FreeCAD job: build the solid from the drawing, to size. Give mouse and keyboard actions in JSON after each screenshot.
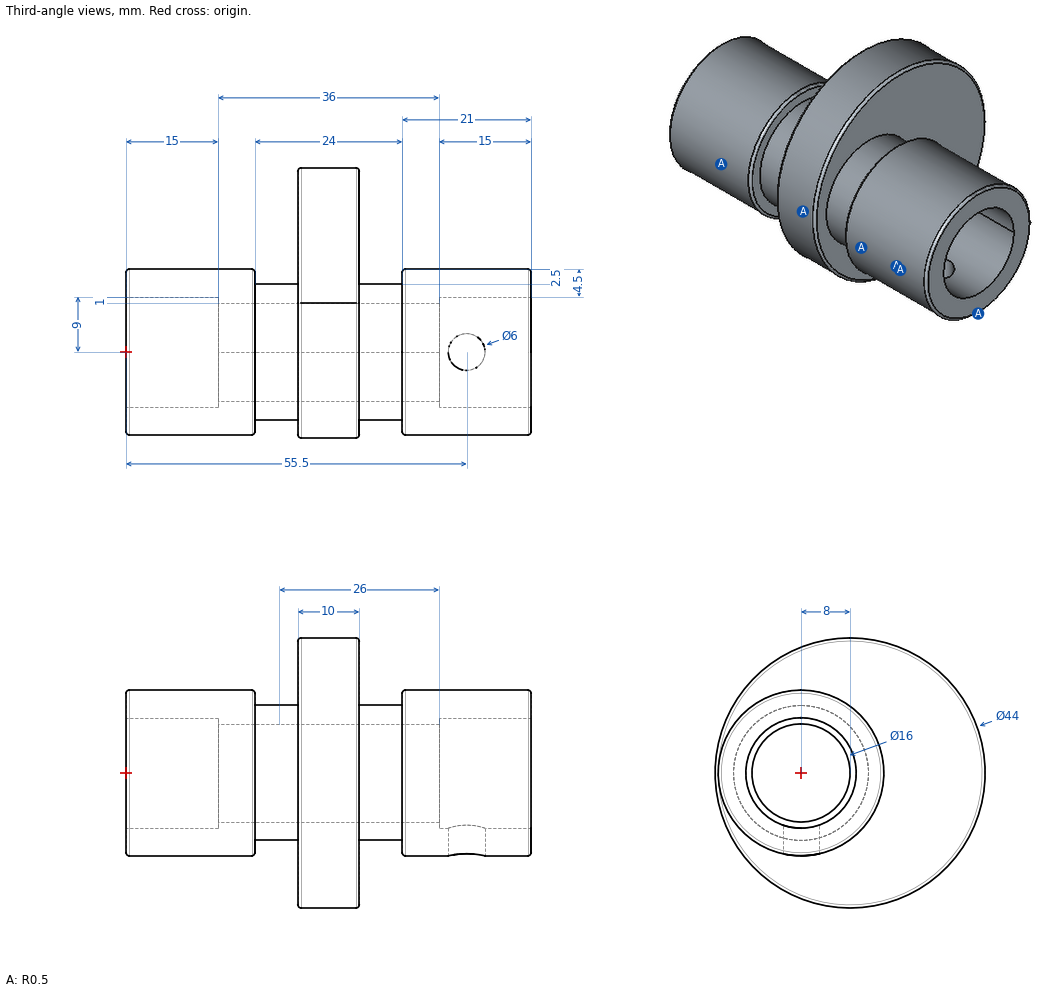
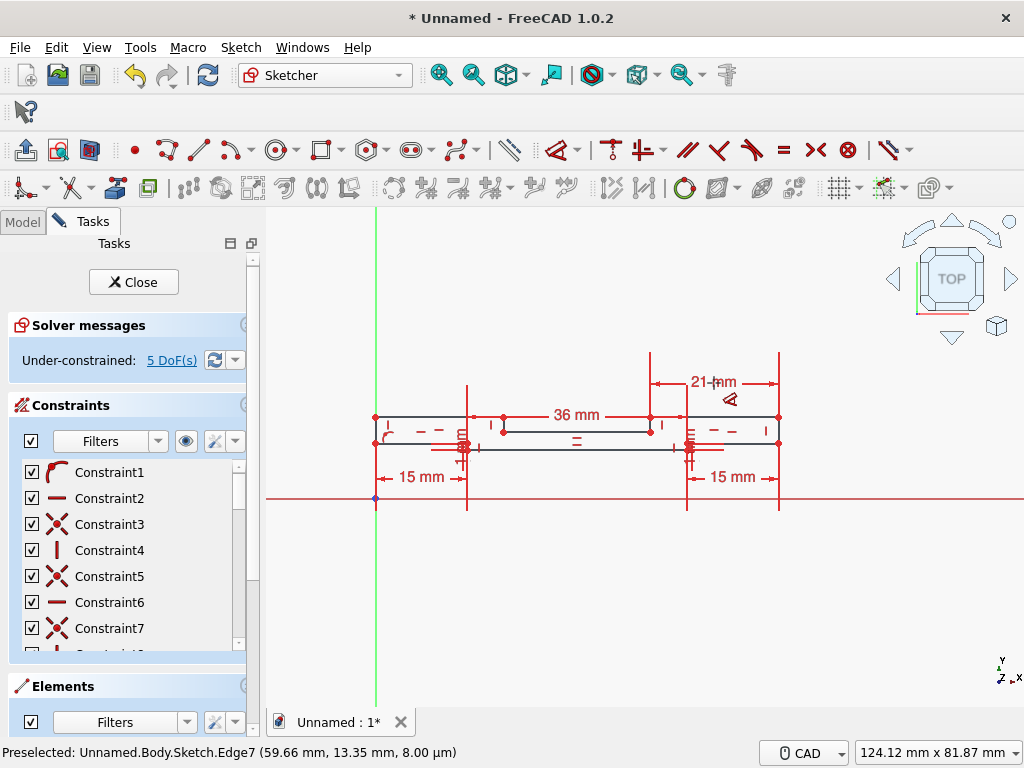
{"action": "left_click", "coordinate": [606, 432]}
{"action": "left_click", "coordinate": [577, 466]}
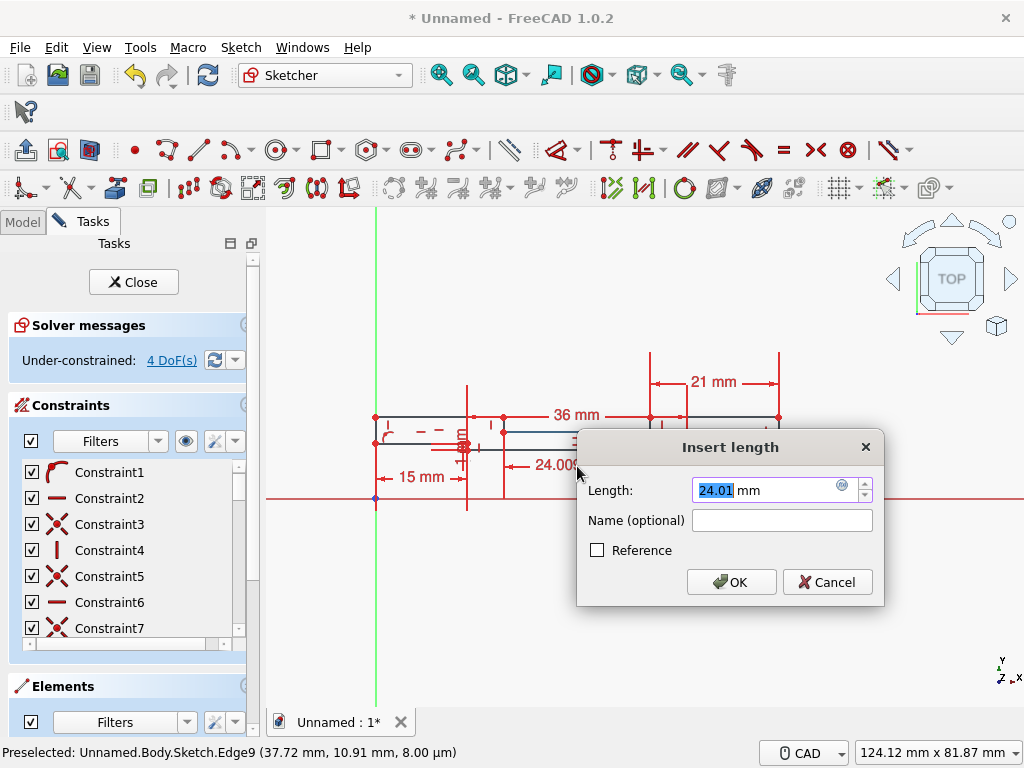
{"action": "type", "text": "24"}
{"action": "key", "text": "Return"}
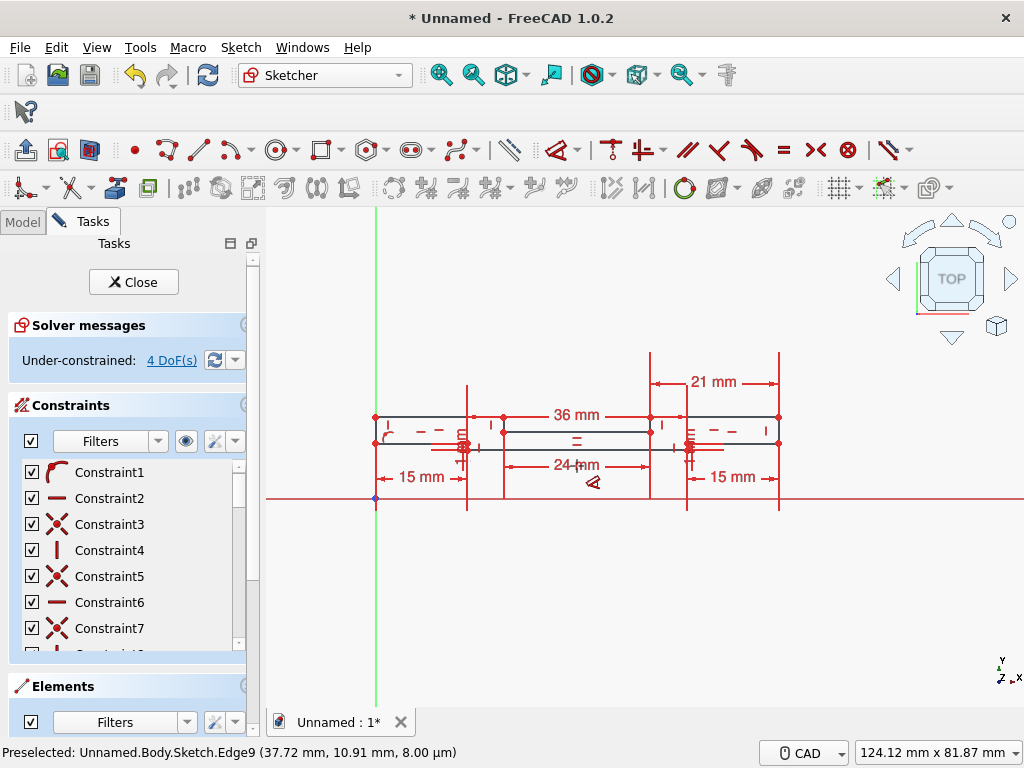
{"action": "left_click", "coordinate": [376, 444]}
{"action": "left_click", "coordinate": [342, 471]}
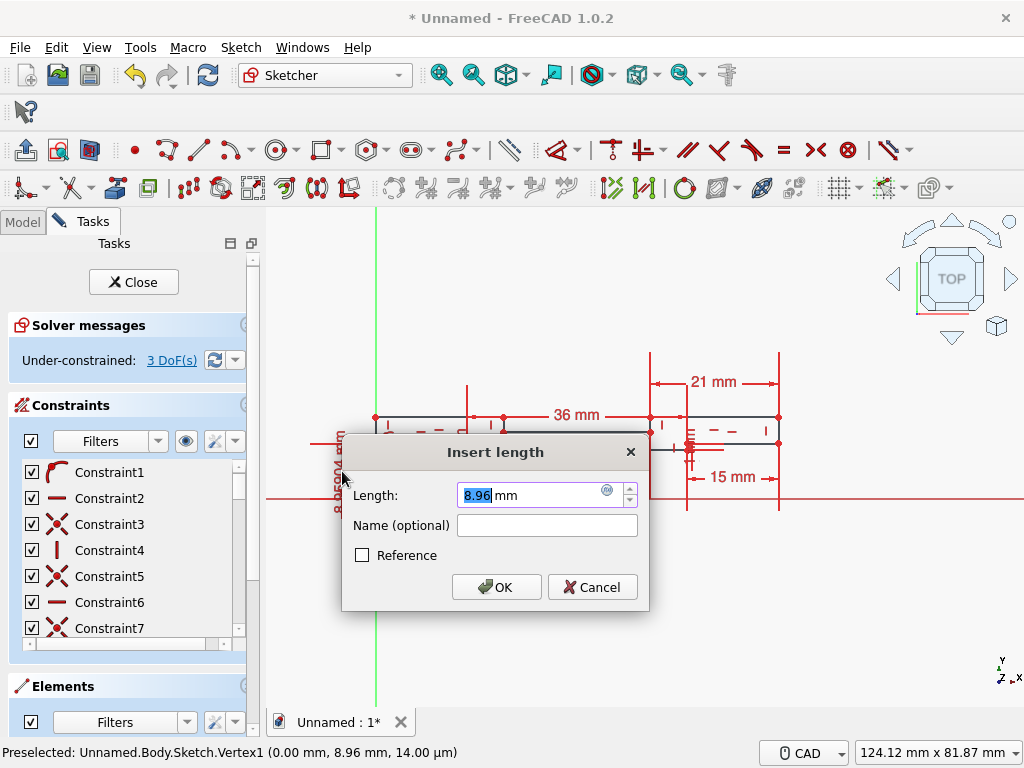
{"action": "type", "text": "9"}
{"action": "key", "text": "Return"}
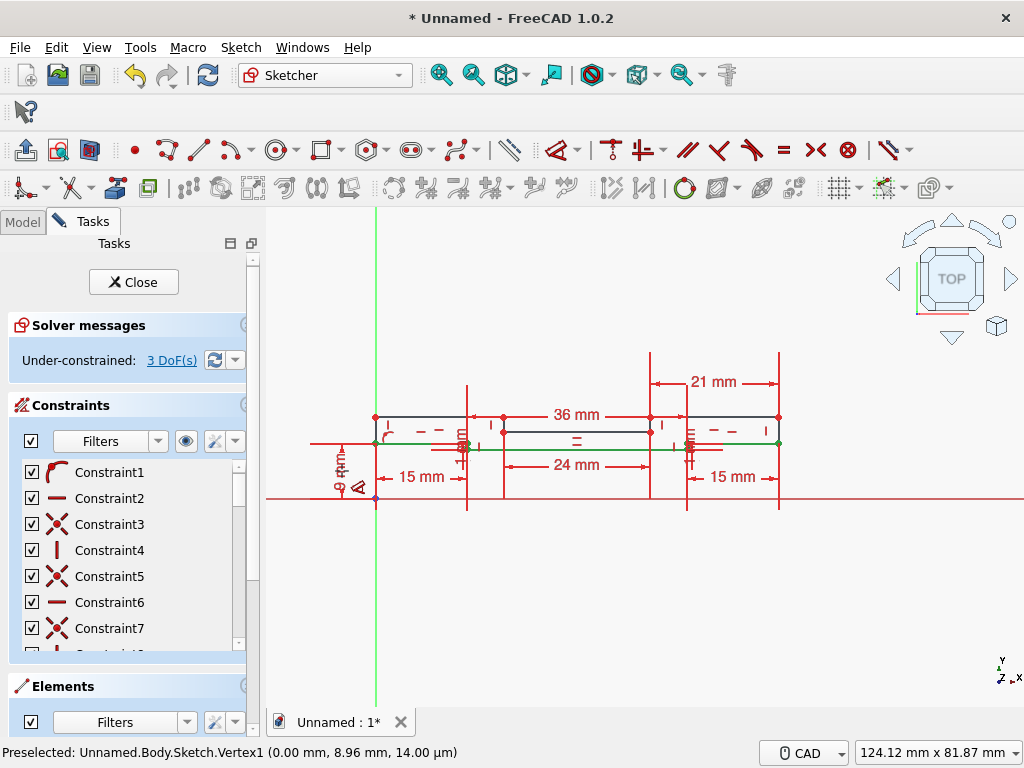
{"action": "scroll", "coordinate": [779, 433], "scroll_direction": "up", "scroll_amount": 2}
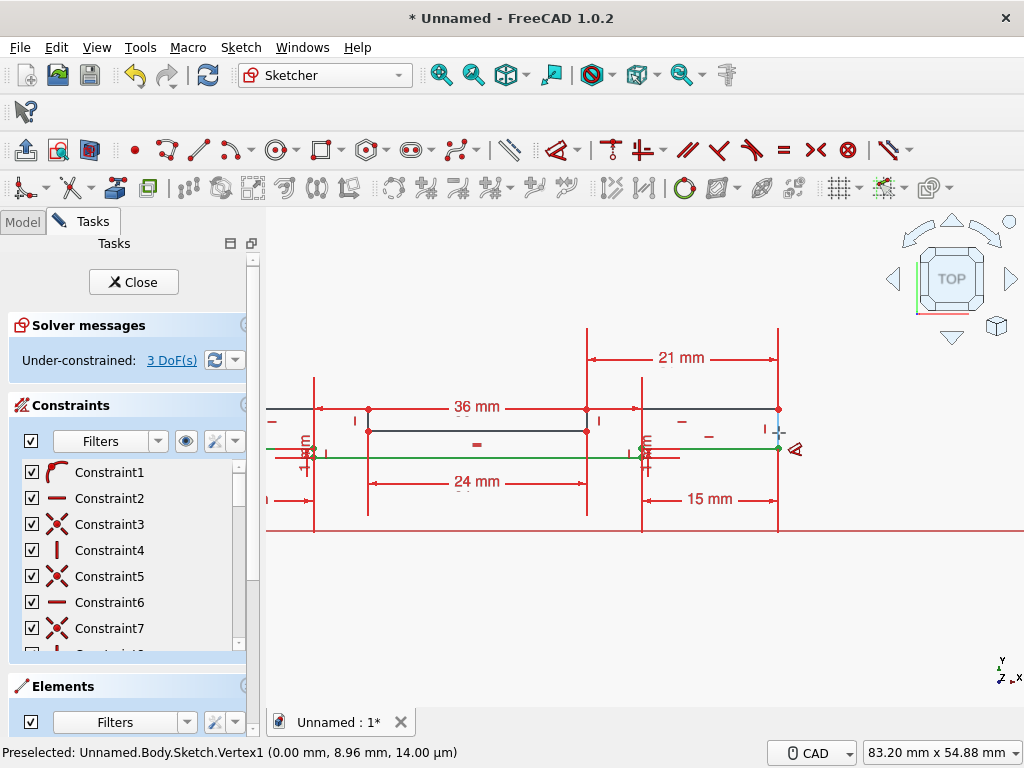
{"action": "left_click", "coordinate": [778, 433]}
{"action": "left_click", "coordinate": [812, 429]}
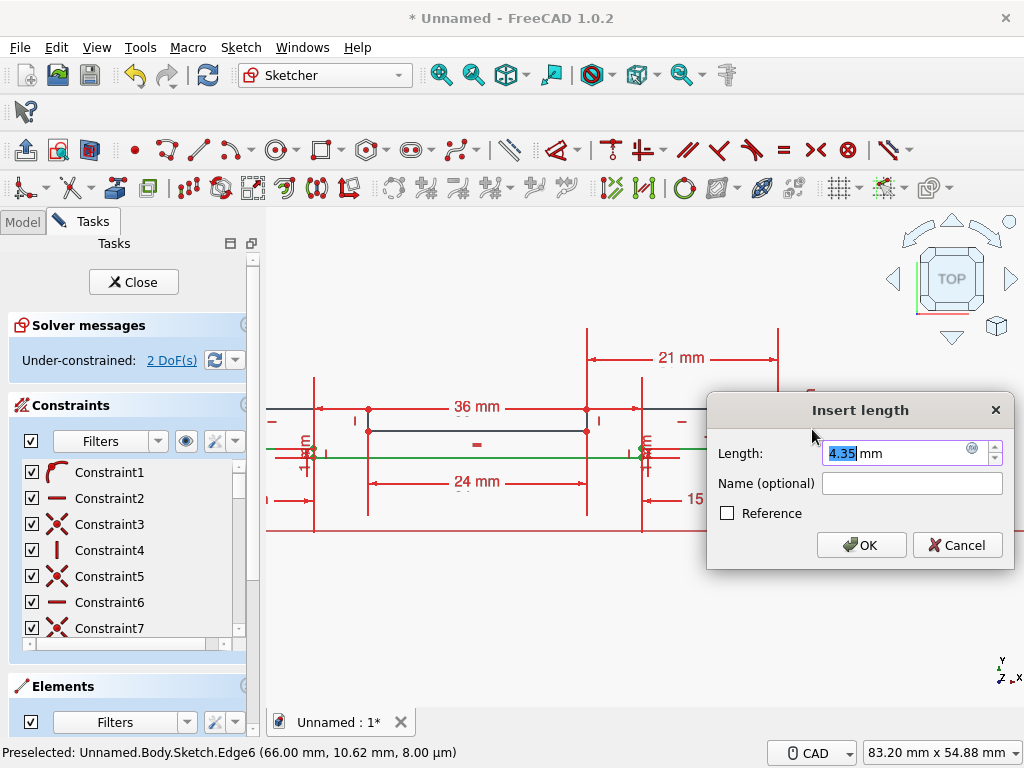
{"action": "type", "text": "4.5"}
{"action": "key", "text": "Return"}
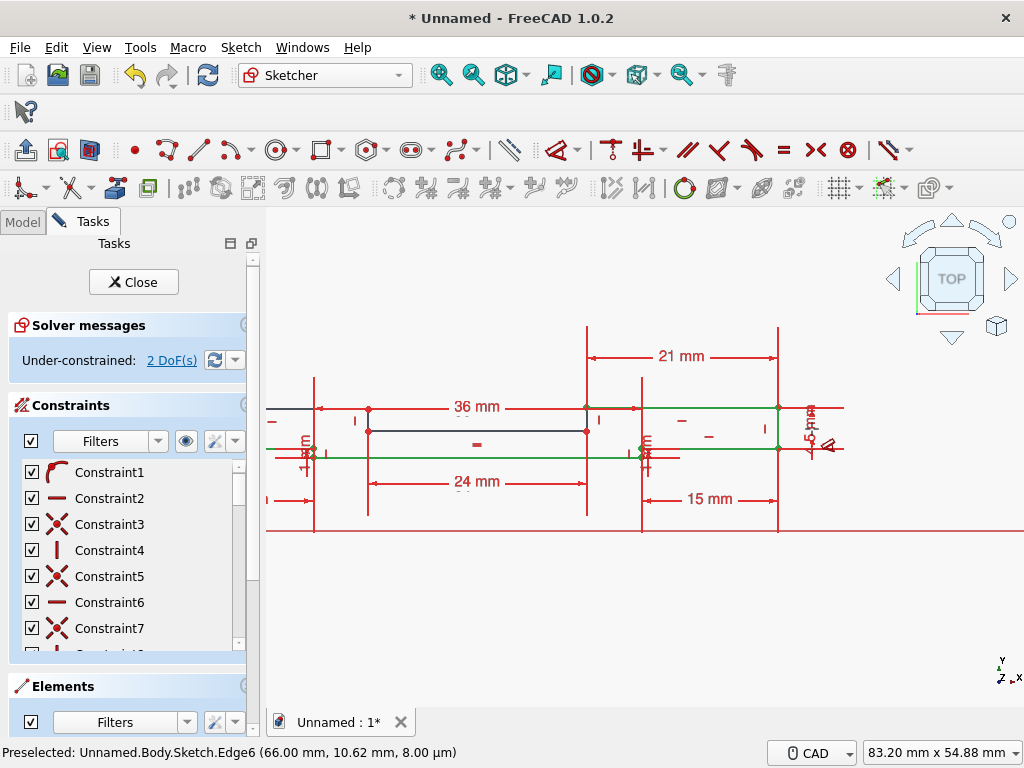
{"action": "scroll", "coordinate": [587, 417], "scroll_direction": "up", "scroll_amount": 3}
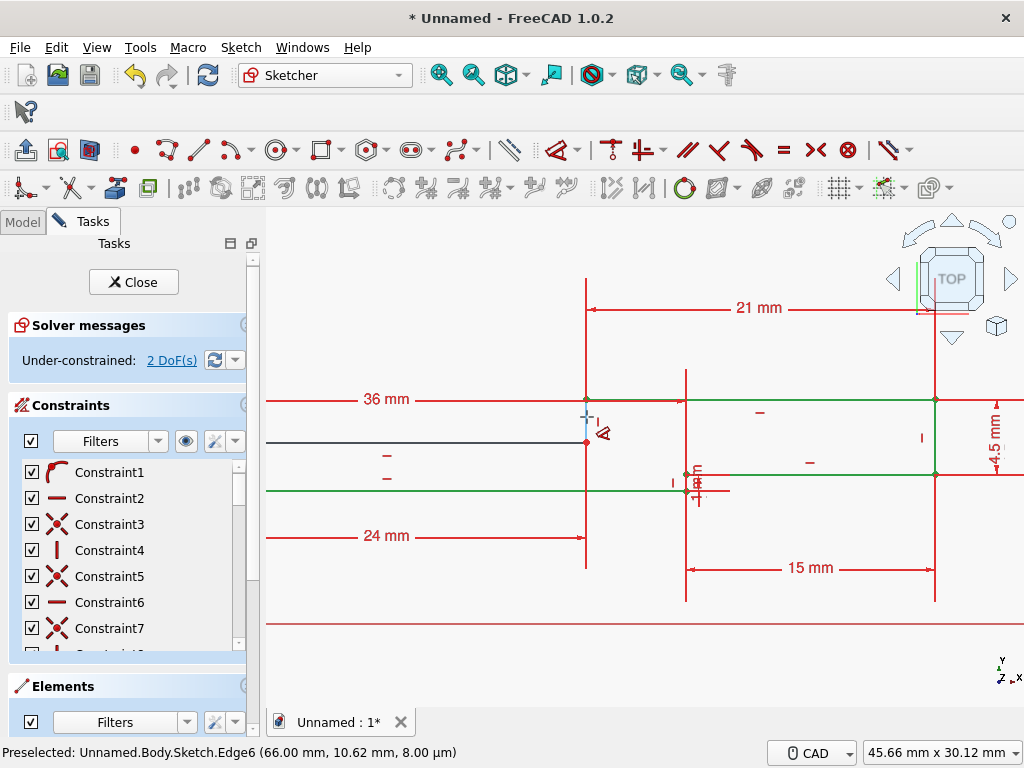
{"action": "left_click", "coordinate": [586, 417]}
{"action": "left_click", "coordinate": [620, 421]}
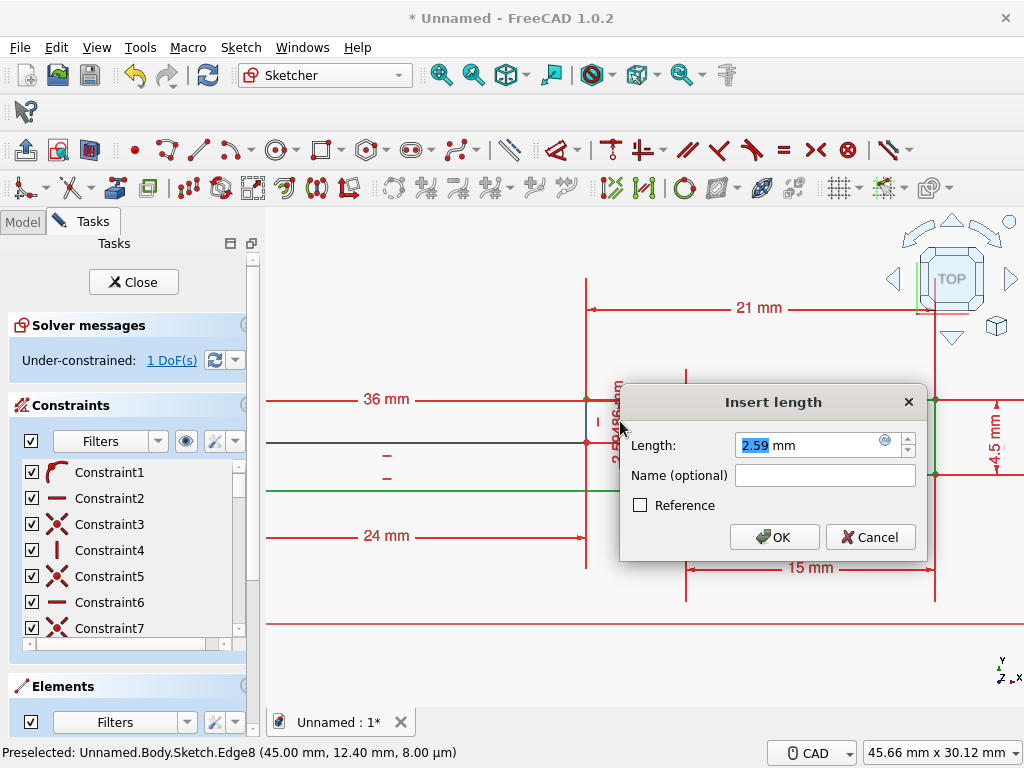
{"action": "type", "text": "2.5"}
{"action": "key", "text": "Return"}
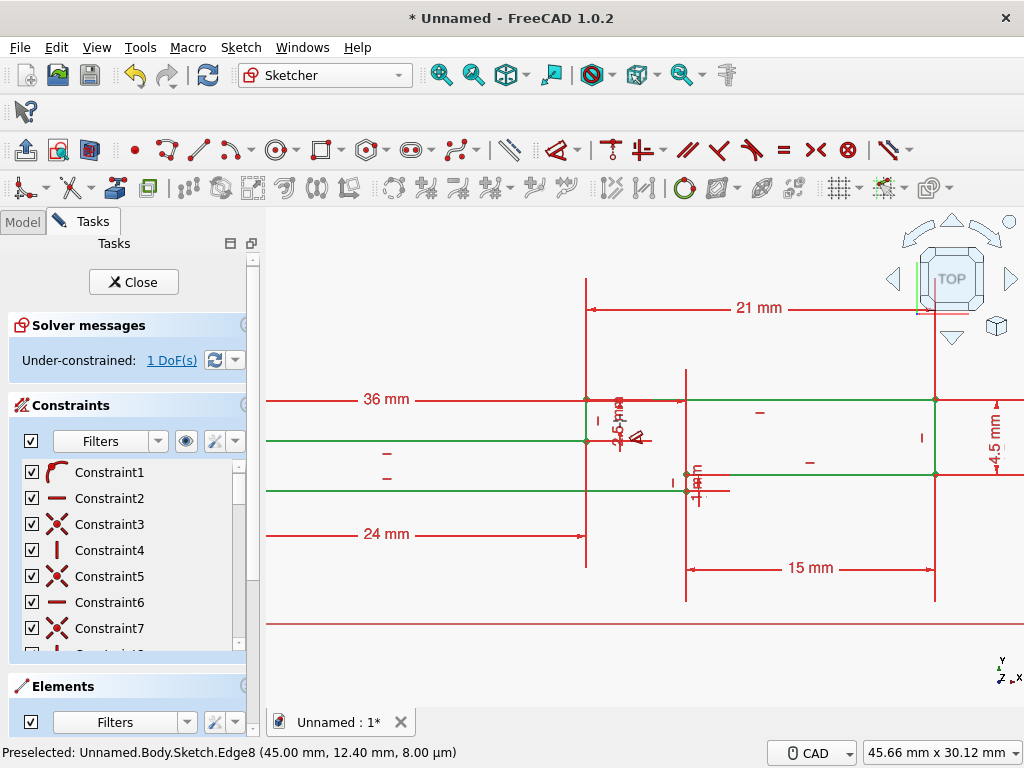
{"action": "scroll", "coordinate": [687, 425], "scroll_direction": "down", "scroll_amount": 5}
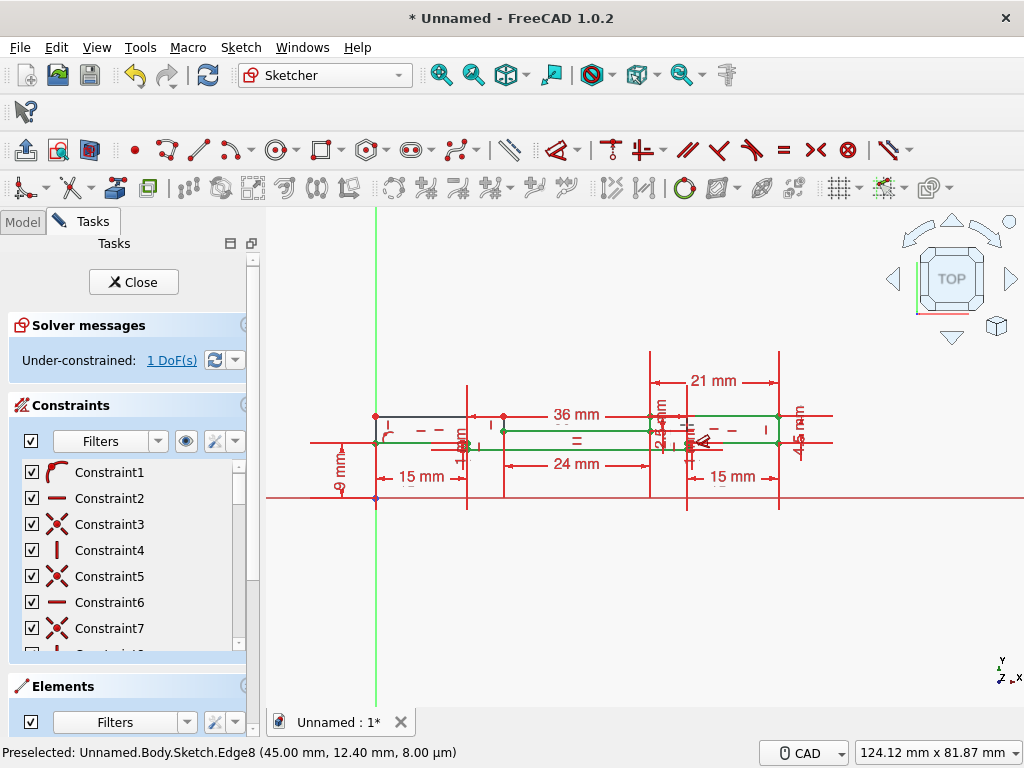
{"action": "scroll", "coordinate": [504, 427], "scroll_direction": "up", "scroll_amount": 6}